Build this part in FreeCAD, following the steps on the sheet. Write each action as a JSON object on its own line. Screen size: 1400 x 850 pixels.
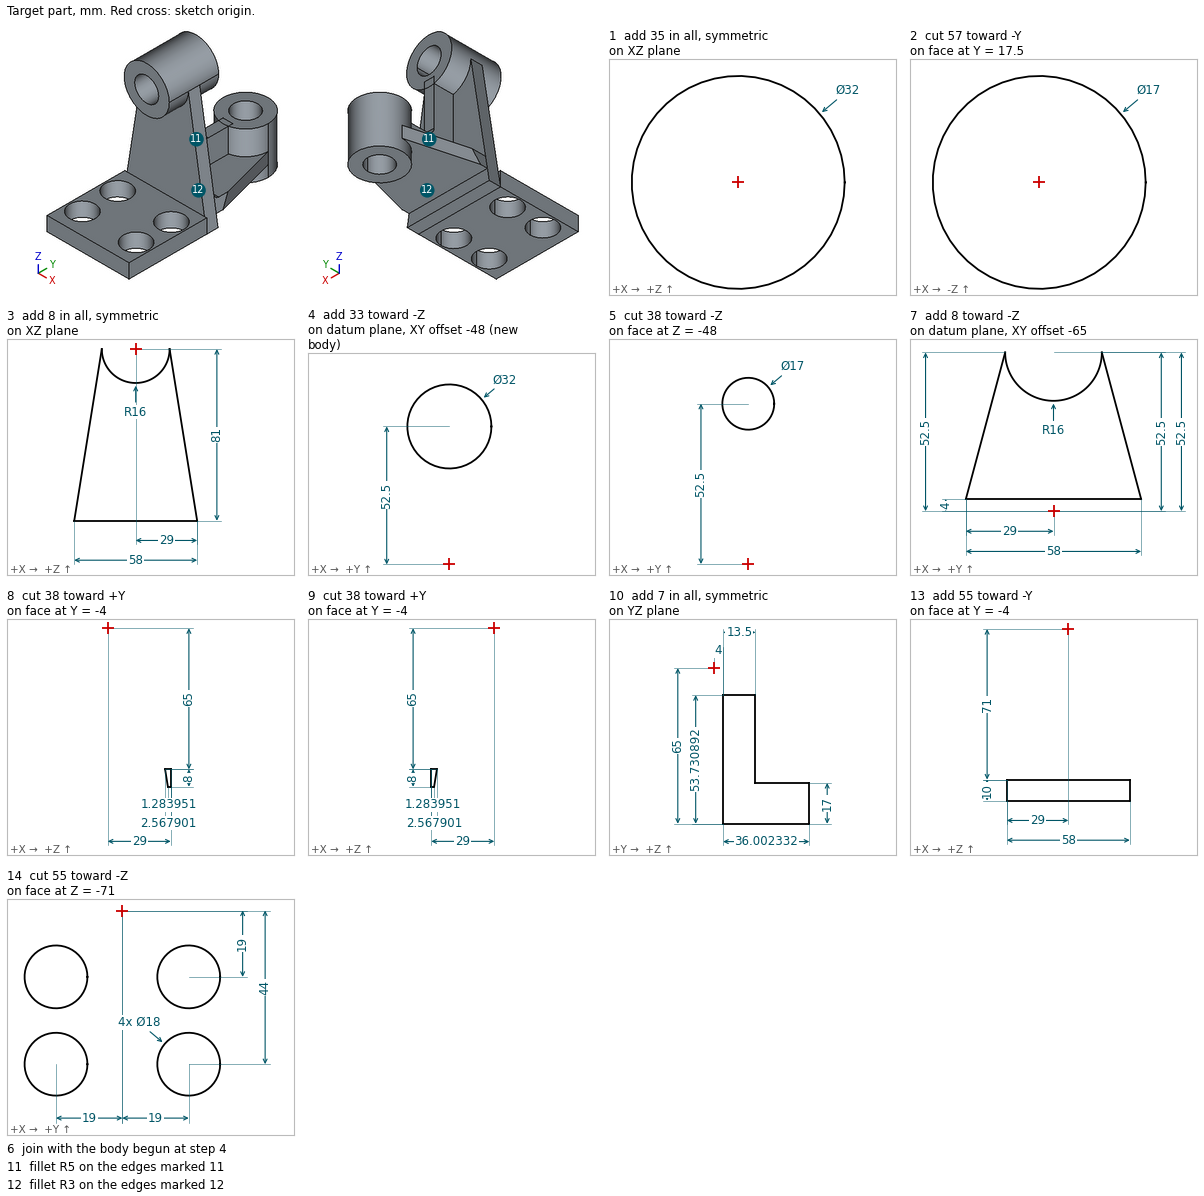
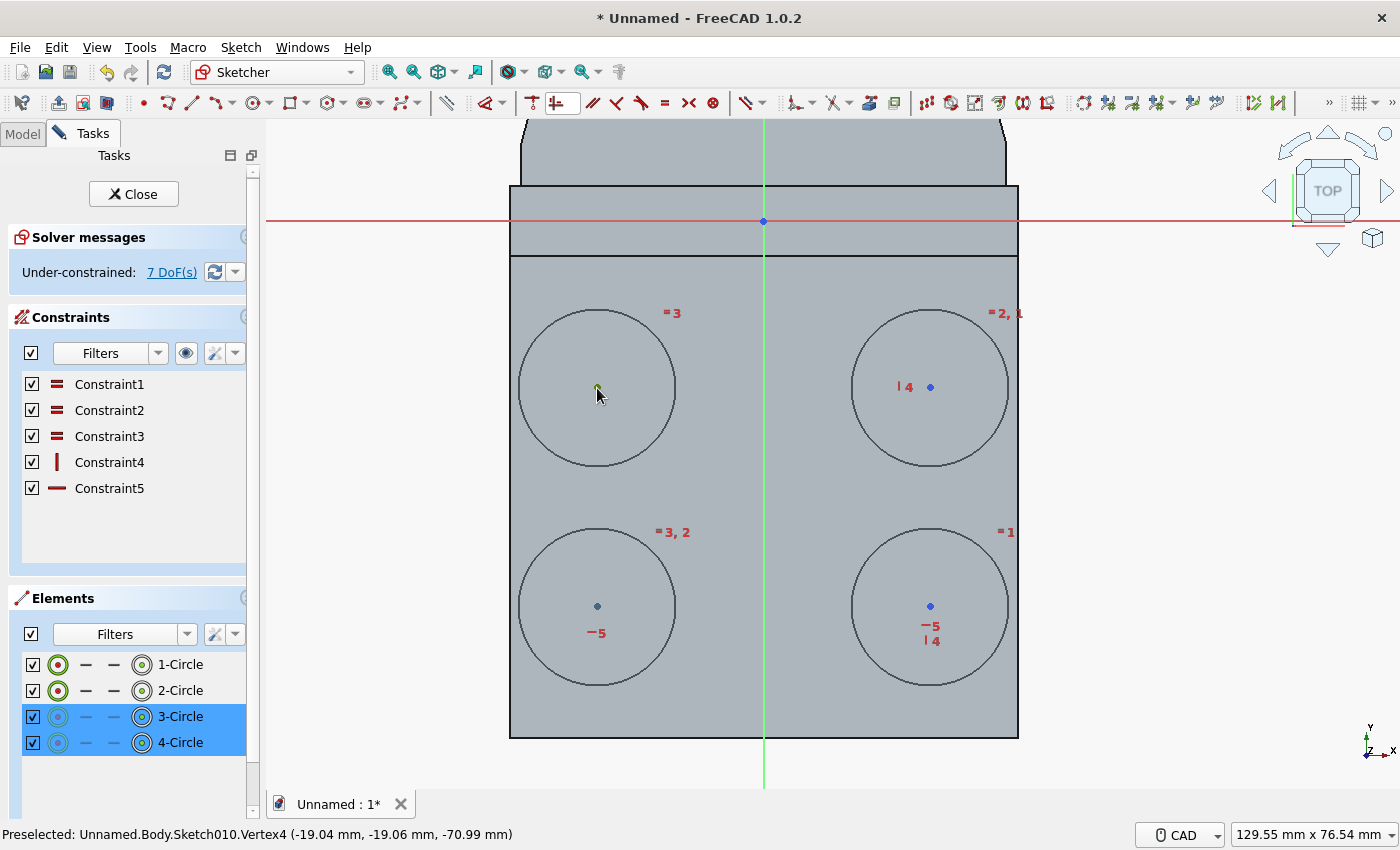
{"action": "key", "text": "v"}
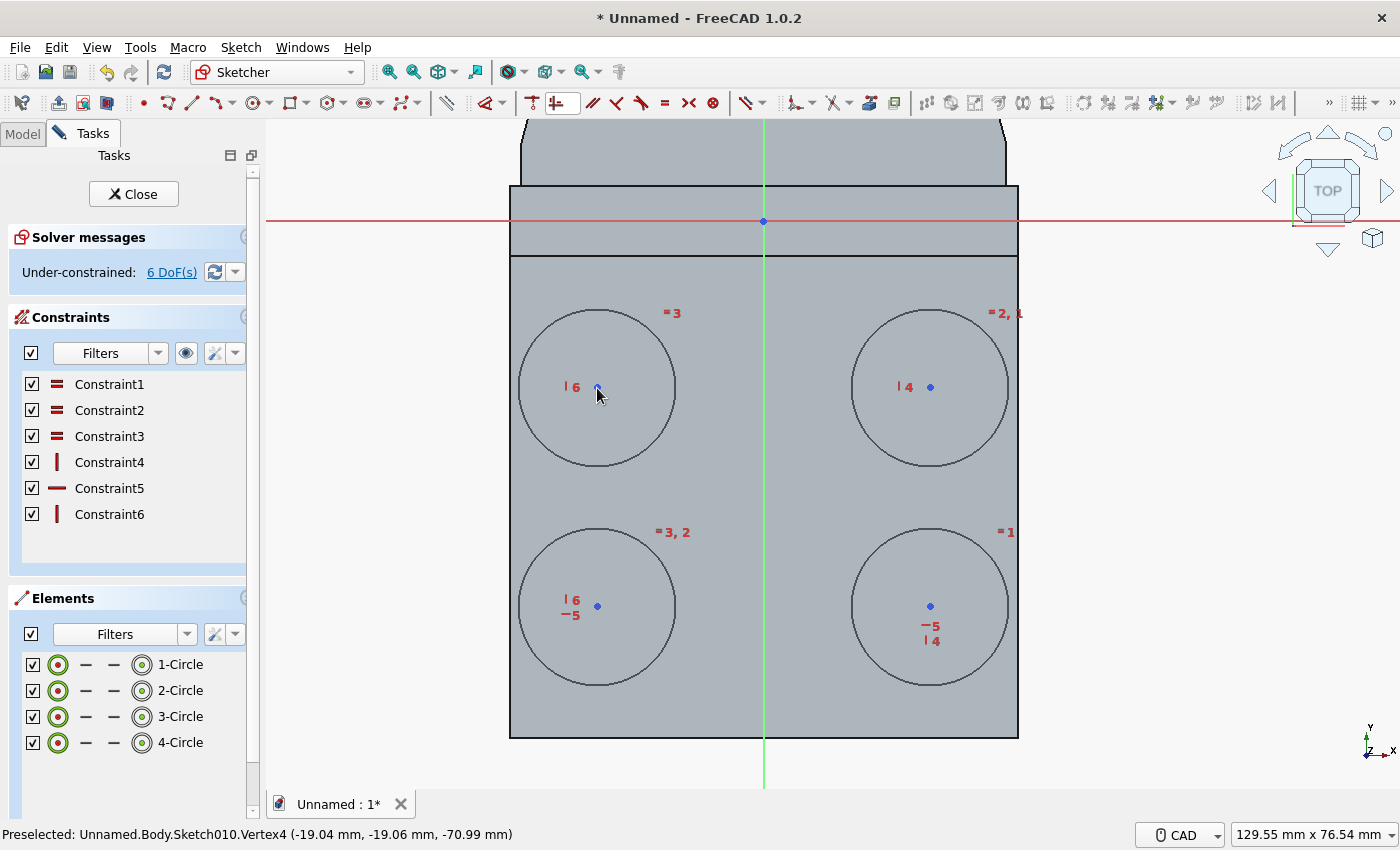
{"action": "left_click", "coordinate": [930, 388]}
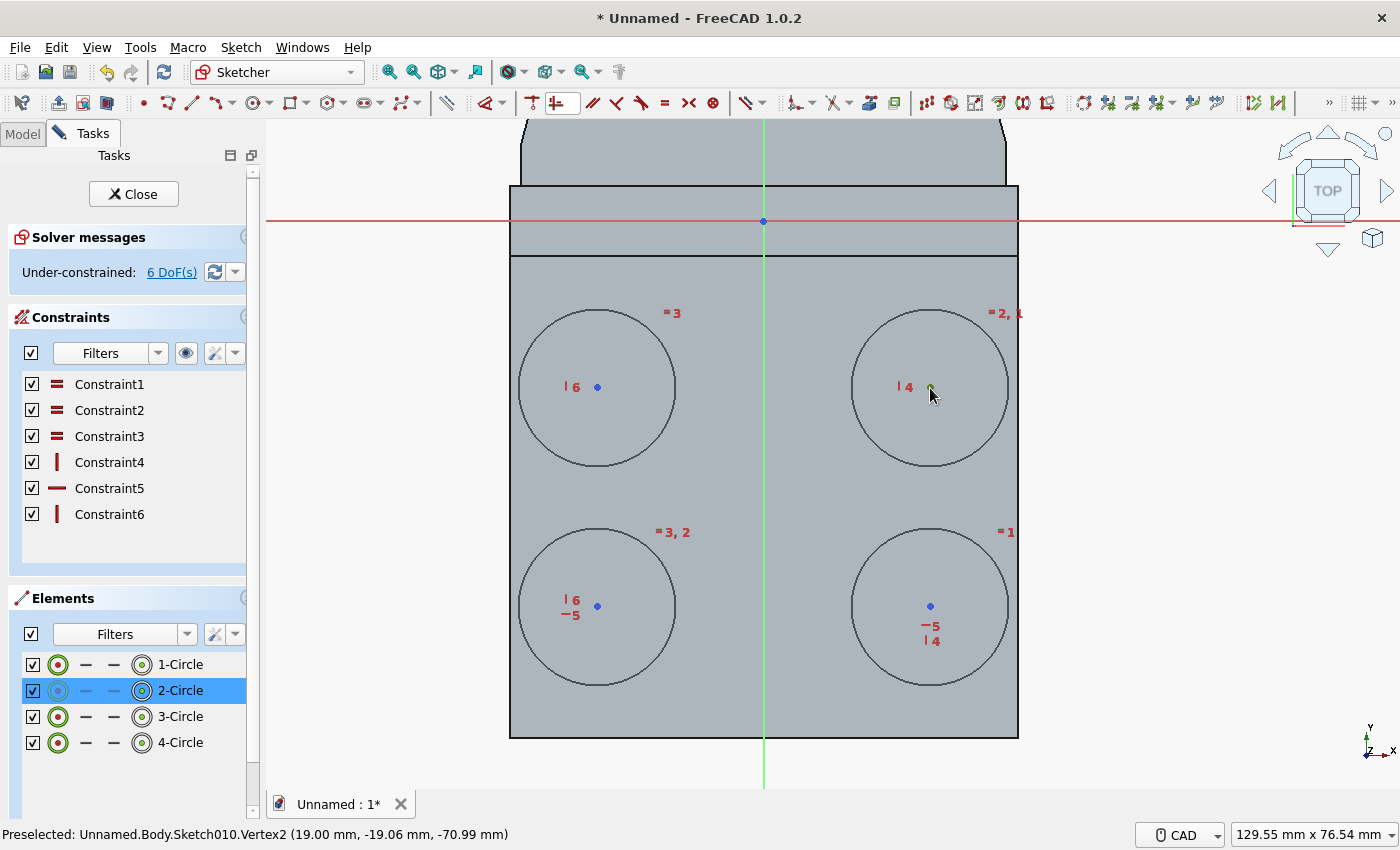
{"action": "left_click", "coordinate": [597, 388]}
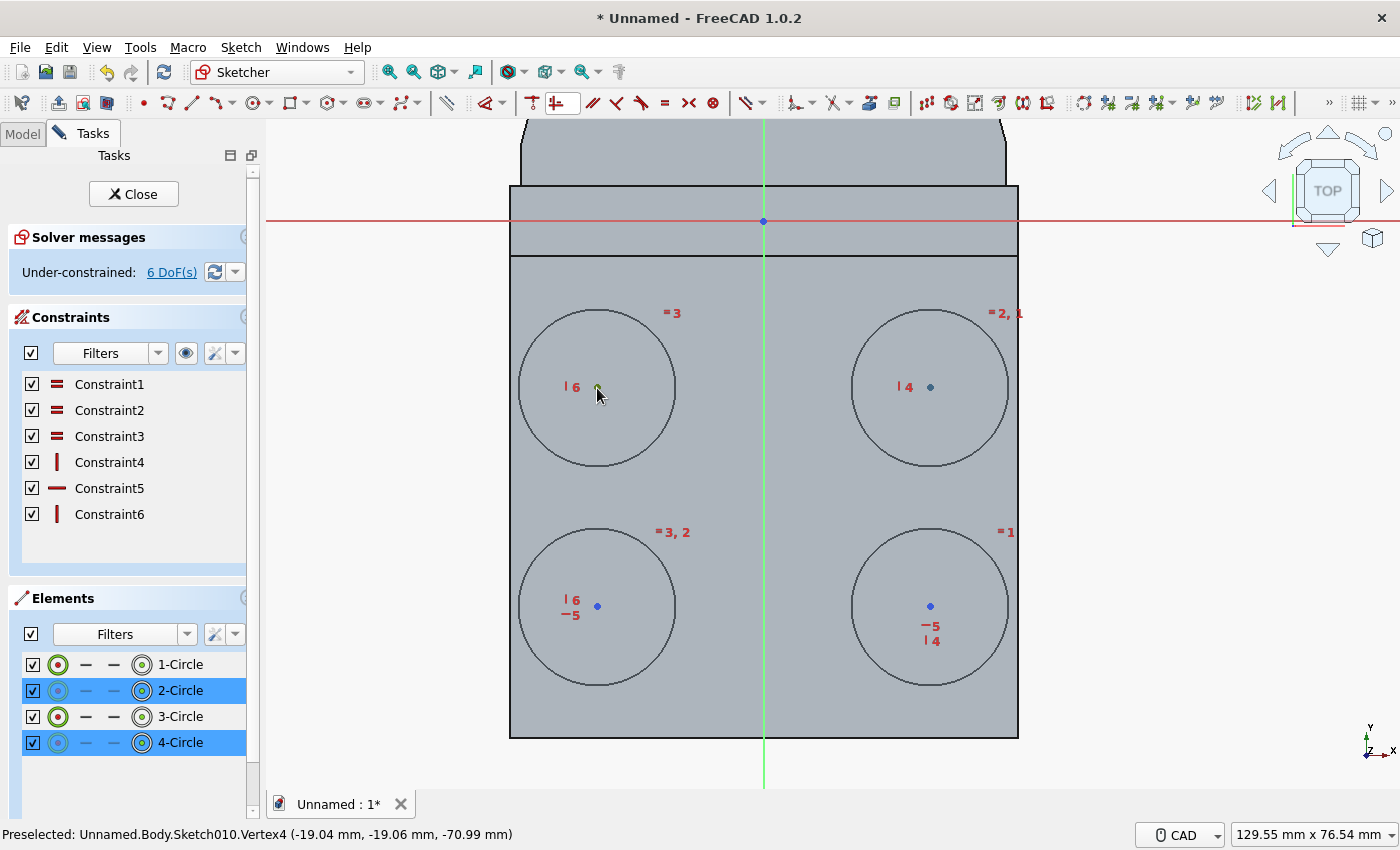
{"action": "key", "text": "h"}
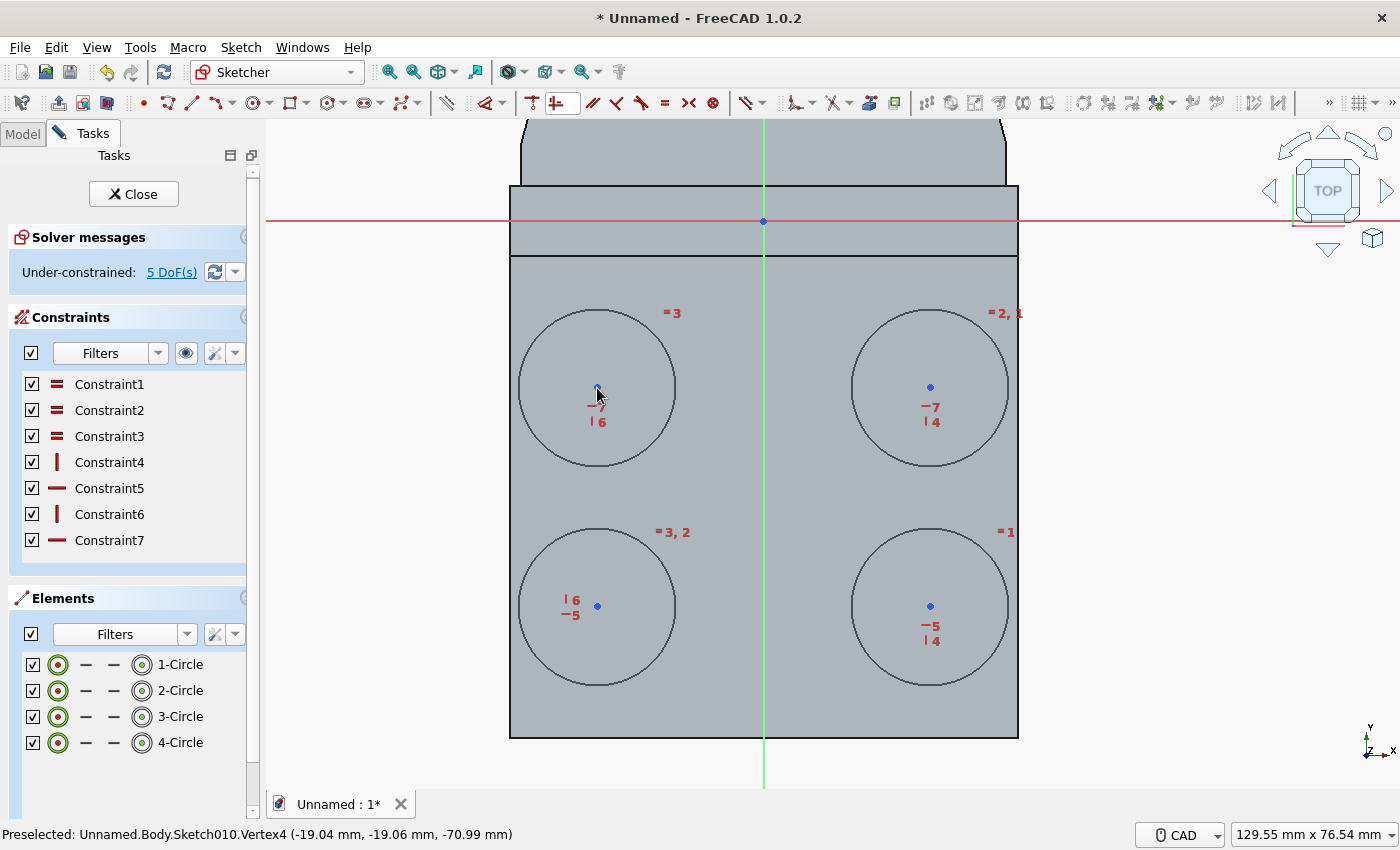
{"action": "key", "text": "d"}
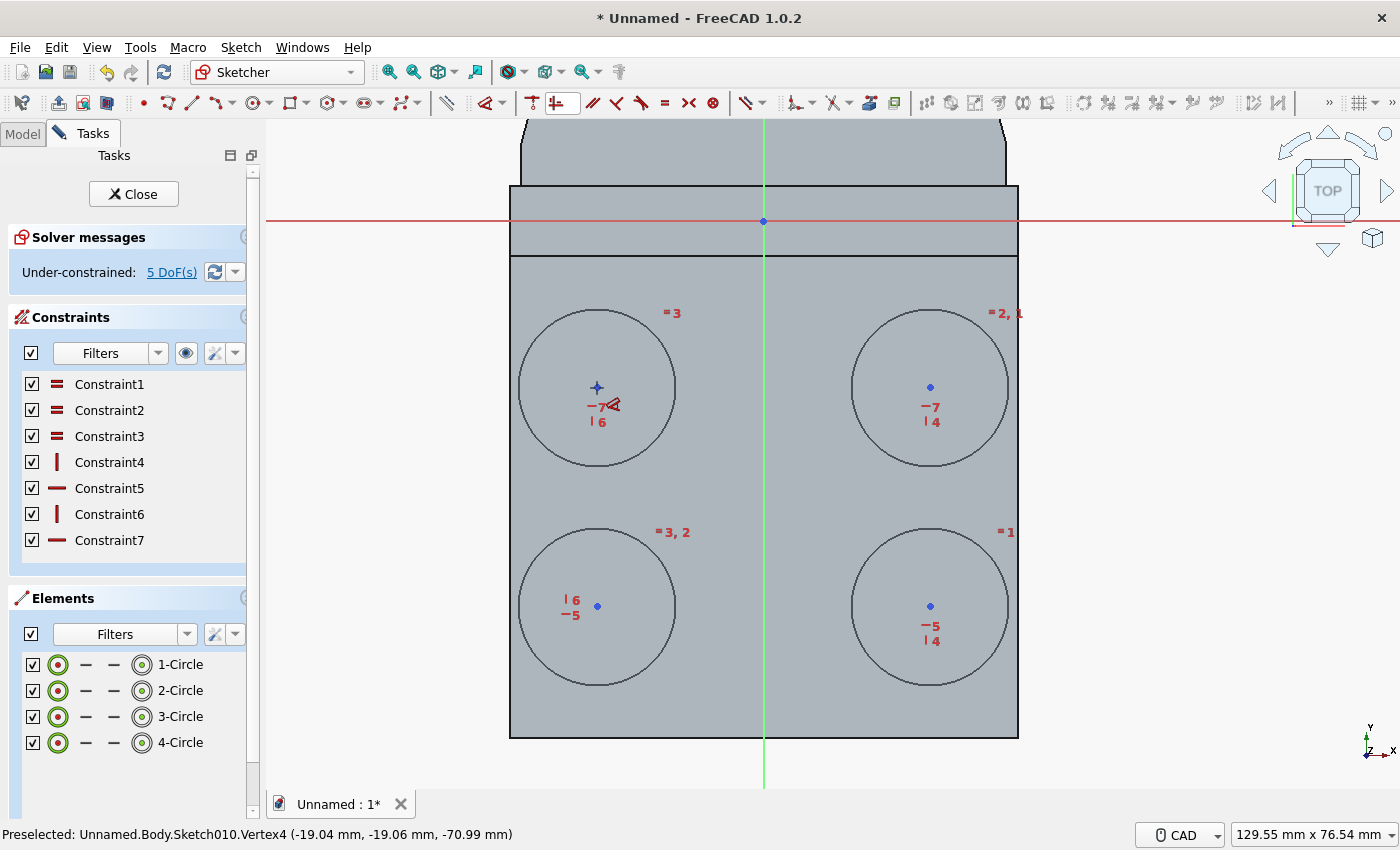
{"action": "left_click", "coordinate": [985, 551]}
{"action": "left_click", "coordinate": [1007, 528]}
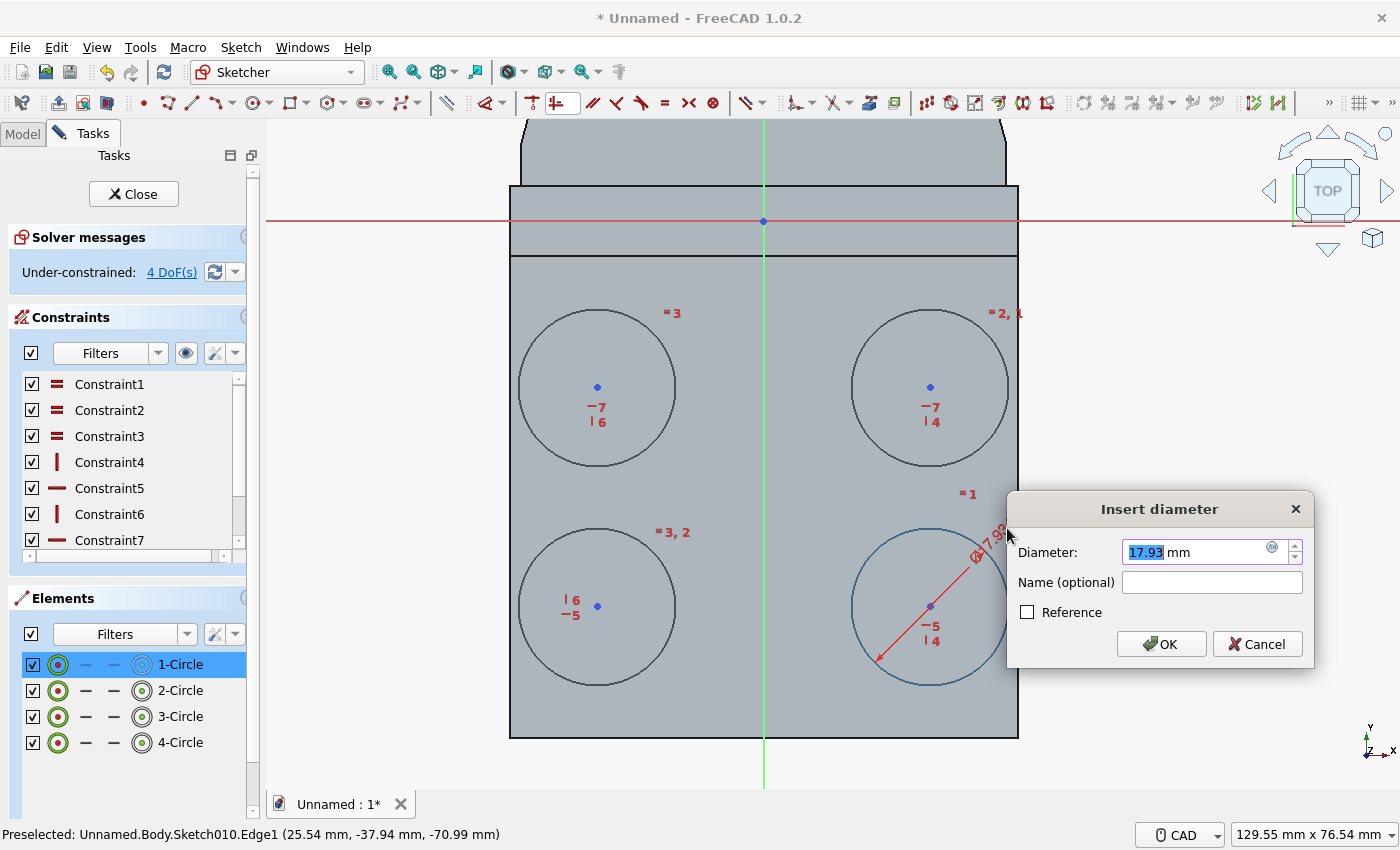
{"action": "type", "text": "18"}
{"action": "key", "text": "Return"}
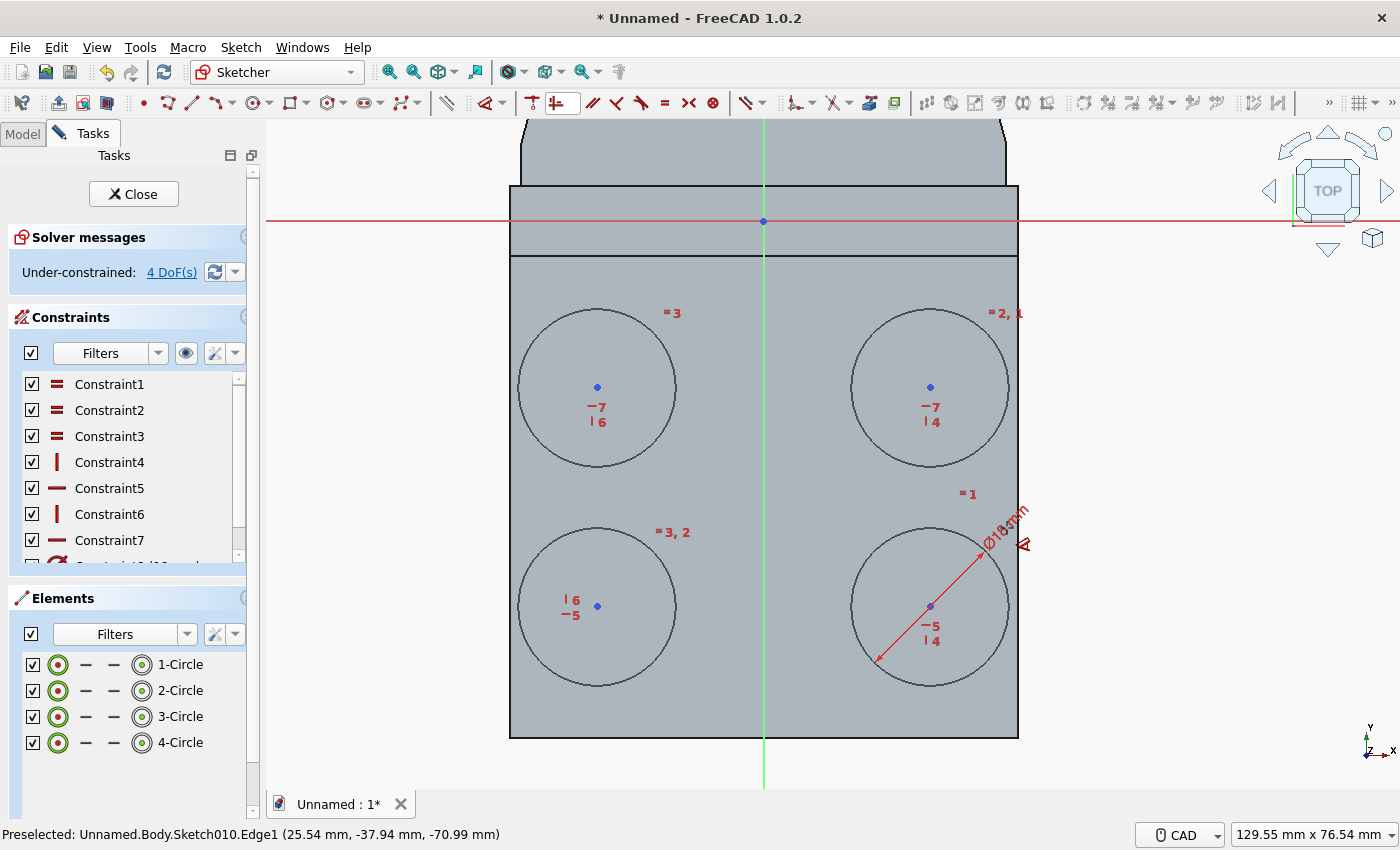
{"action": "left_click", "coordinate": [930, 607]}
{"action": "left_click", "coordinate": [847, 187]}